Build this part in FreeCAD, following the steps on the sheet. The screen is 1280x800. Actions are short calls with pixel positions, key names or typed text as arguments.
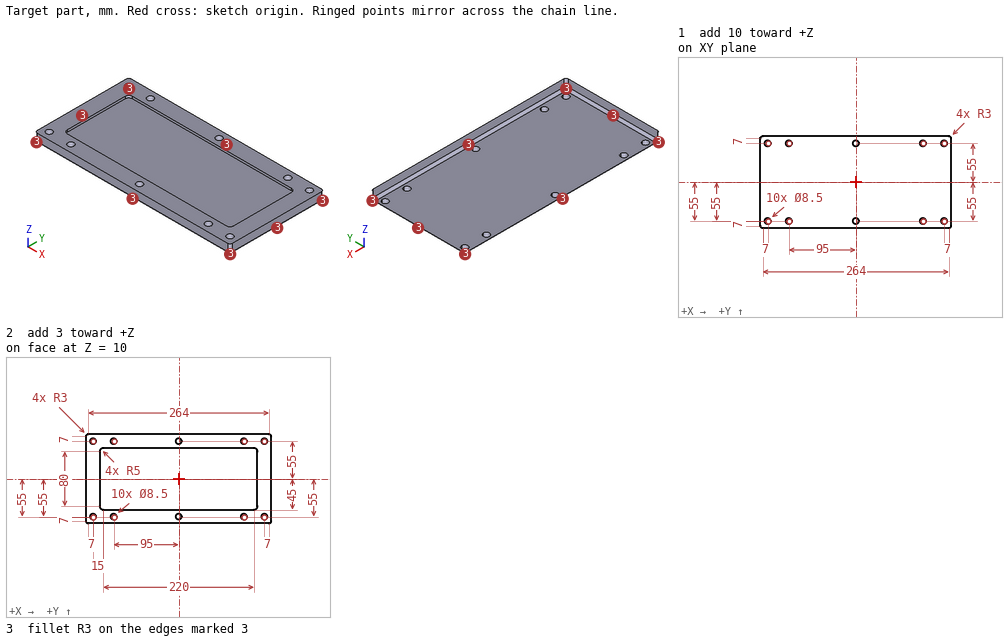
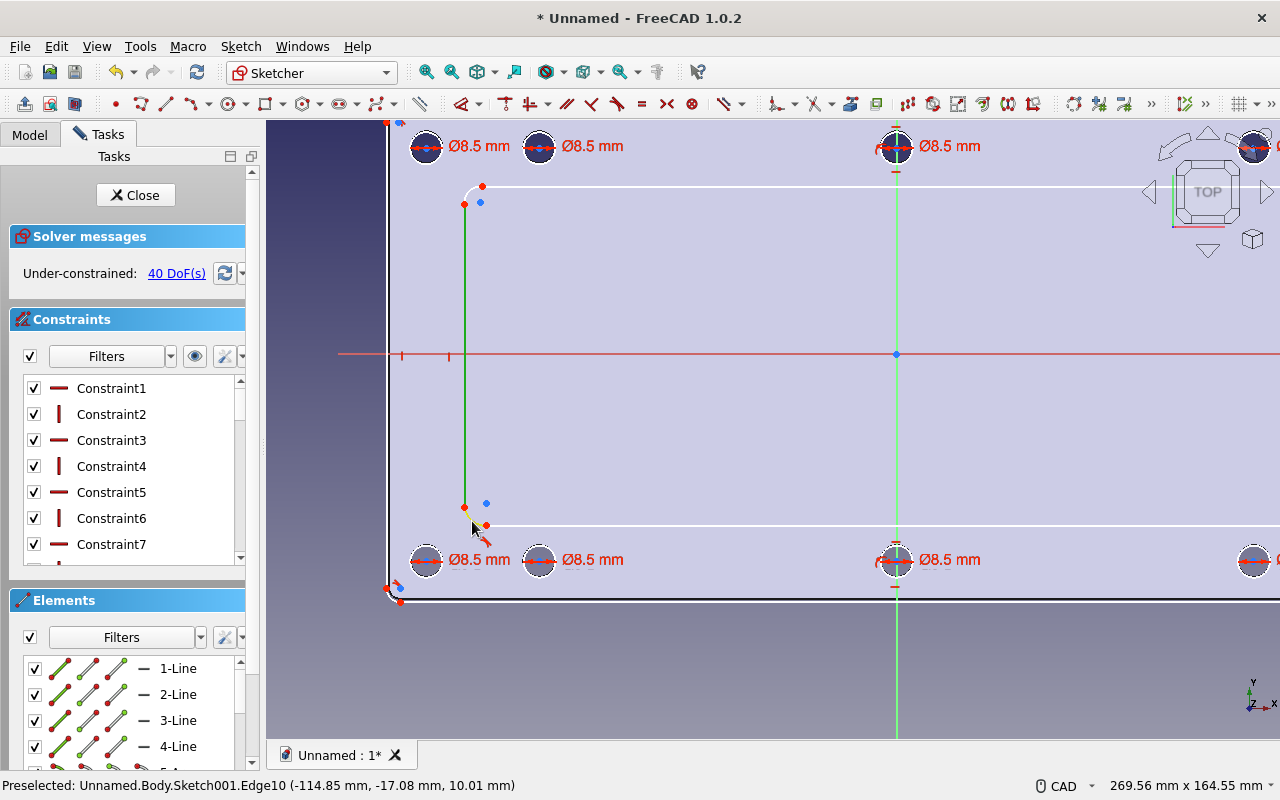
click(472, 521)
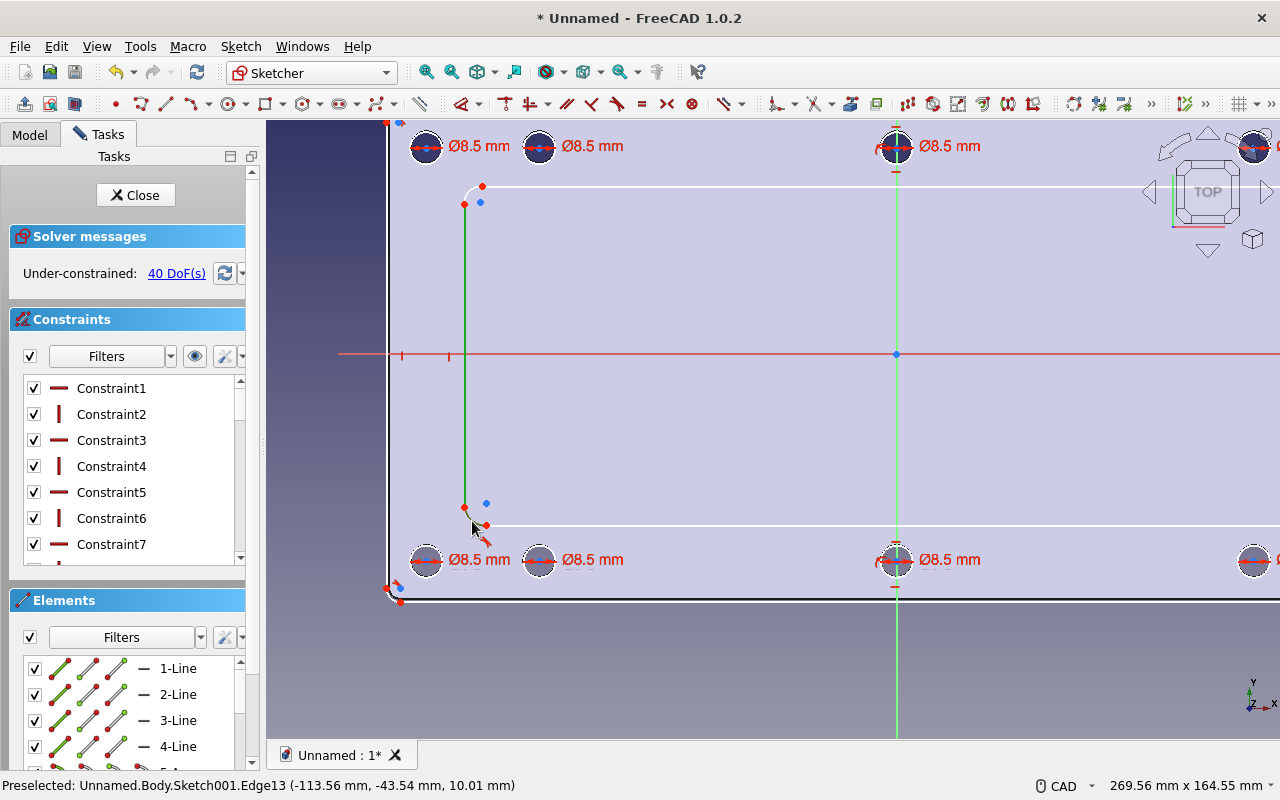
click(617, 104)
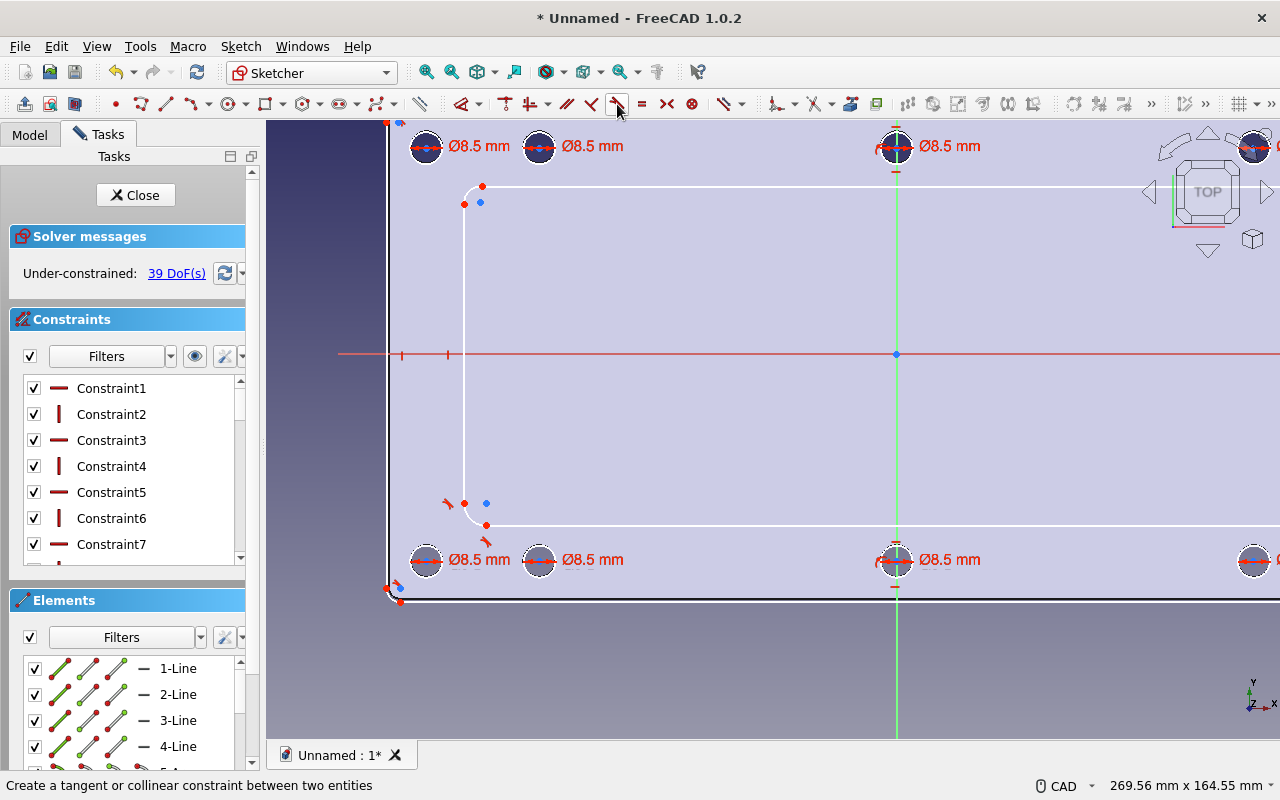
click(464, 414)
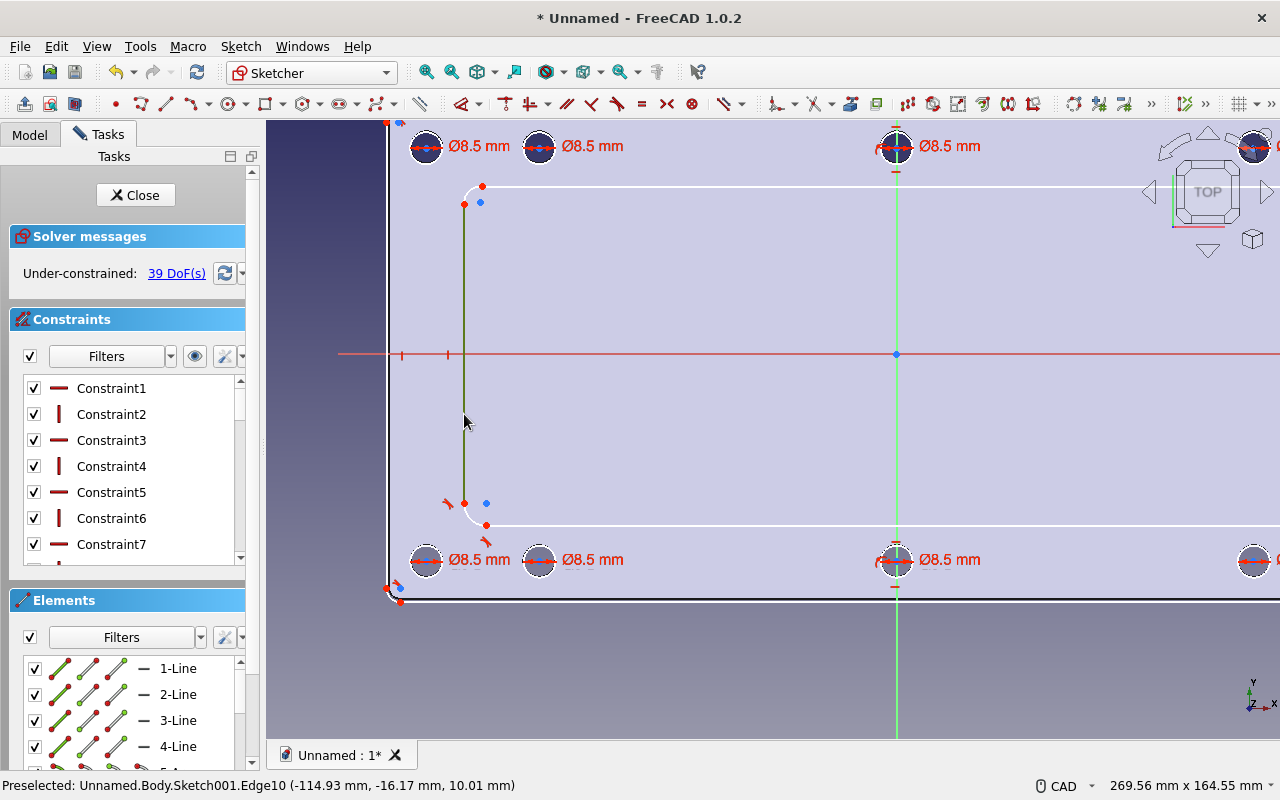
click(469, 191)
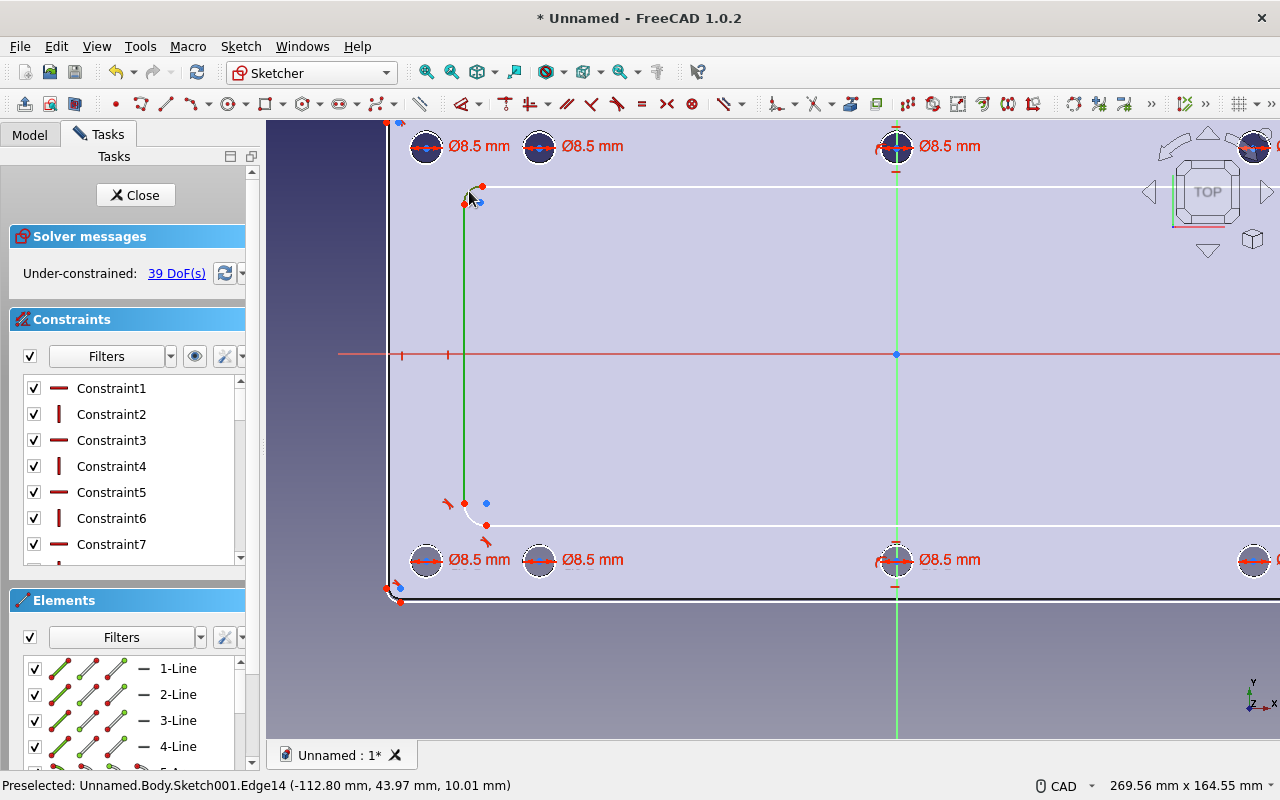
click(617, 104)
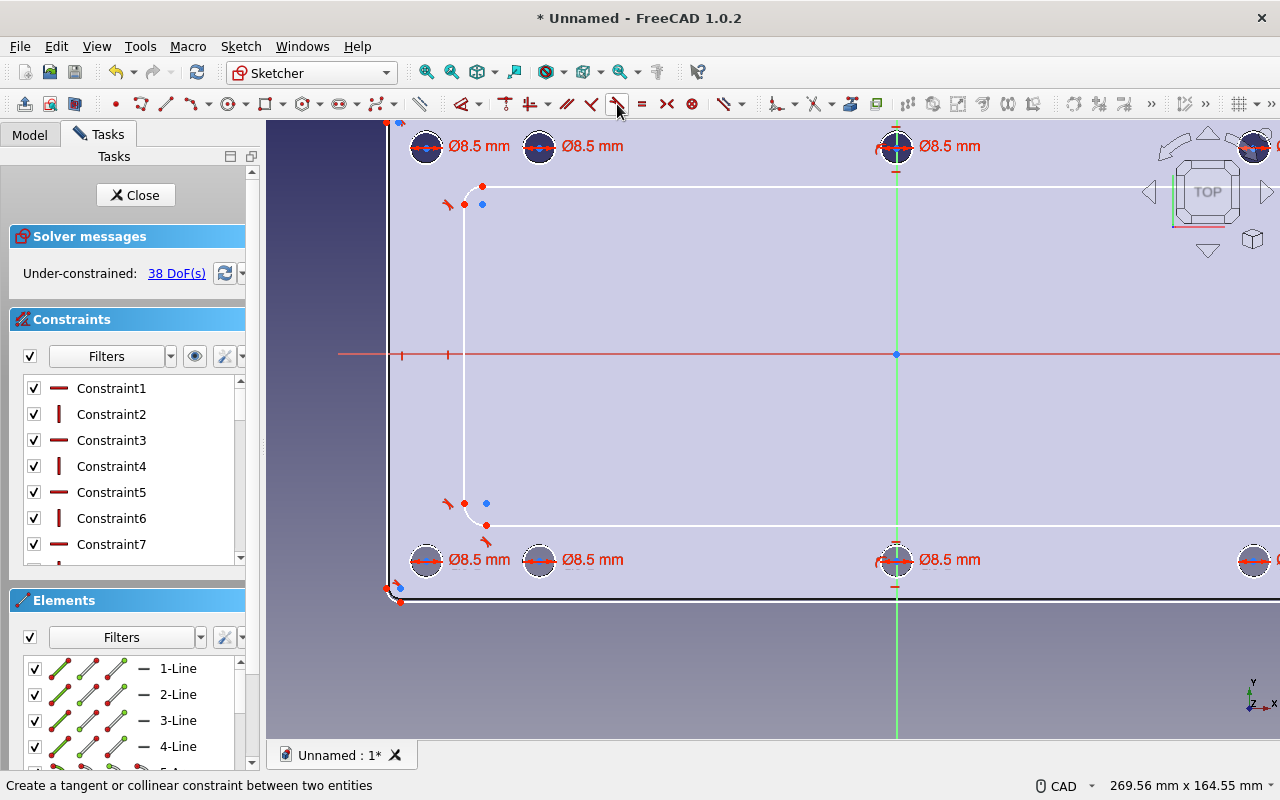
click(731, 187)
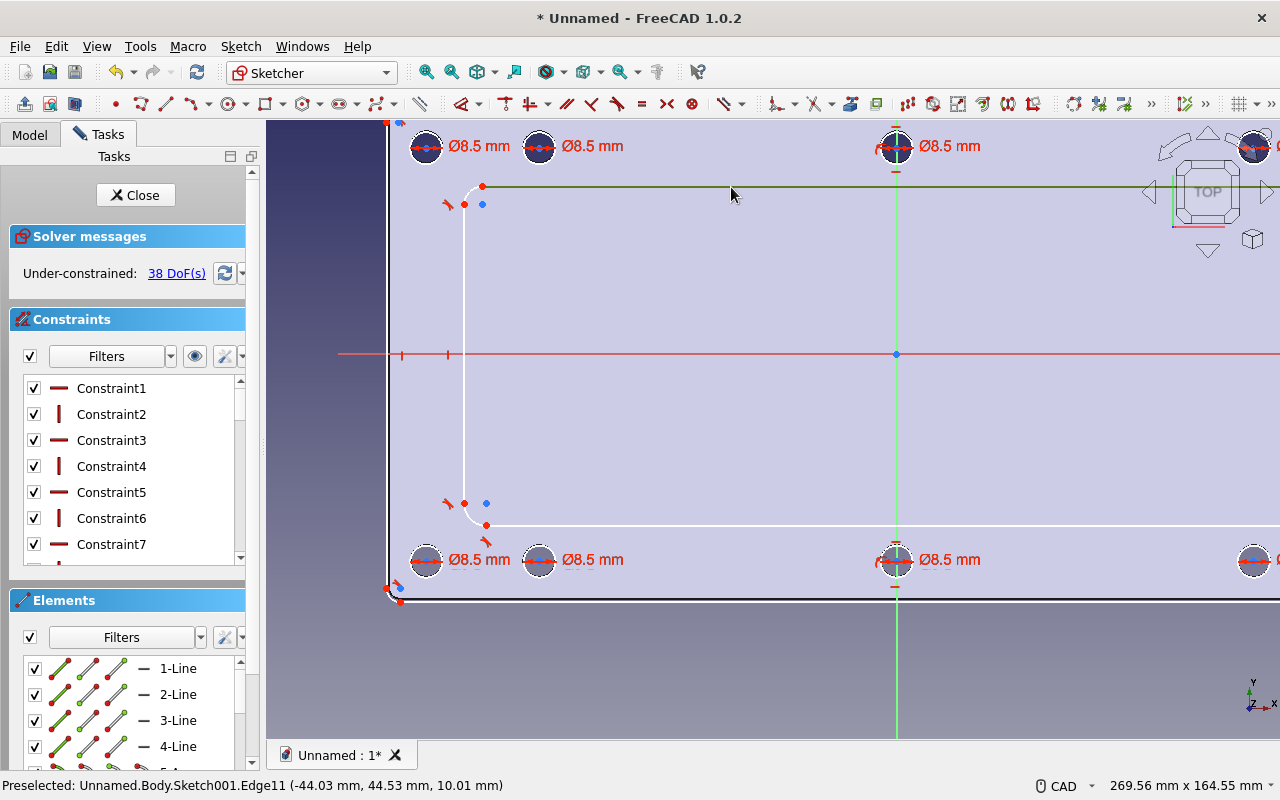
click(470, 192)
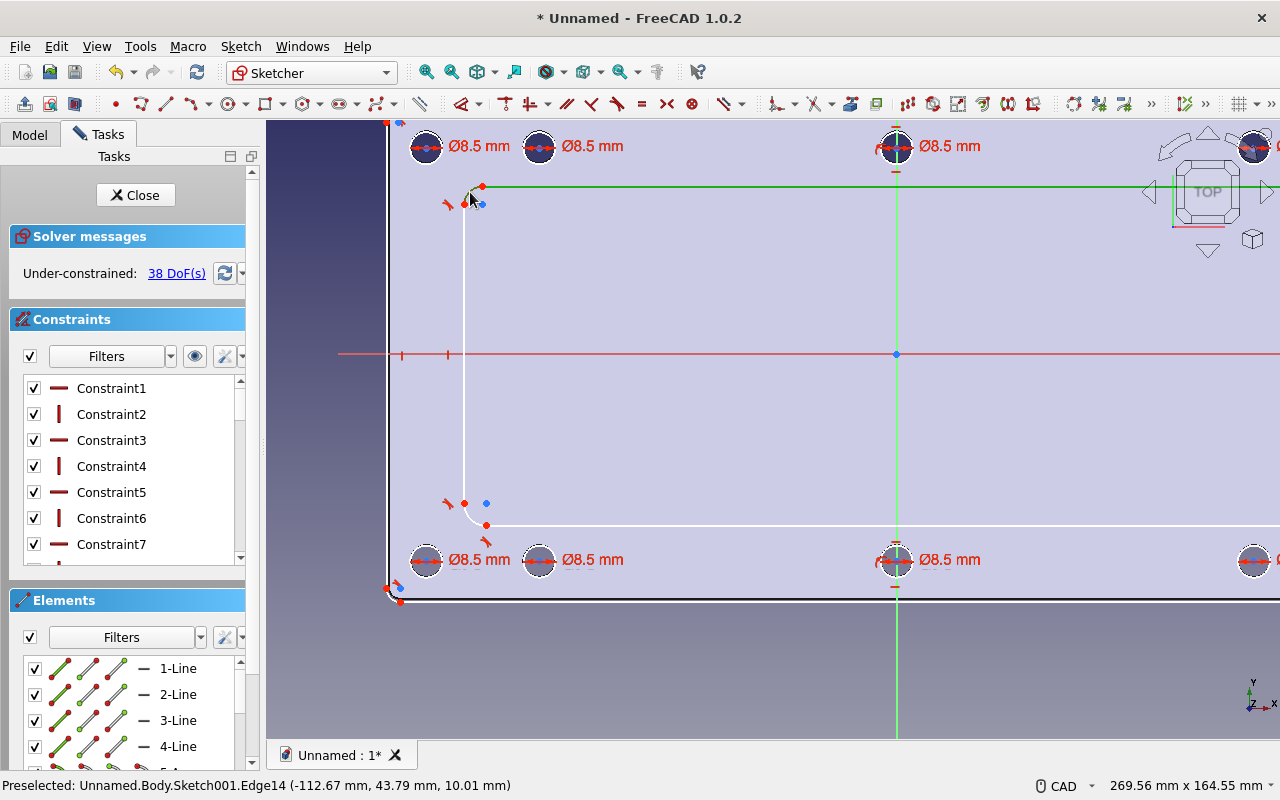
click(617, 104)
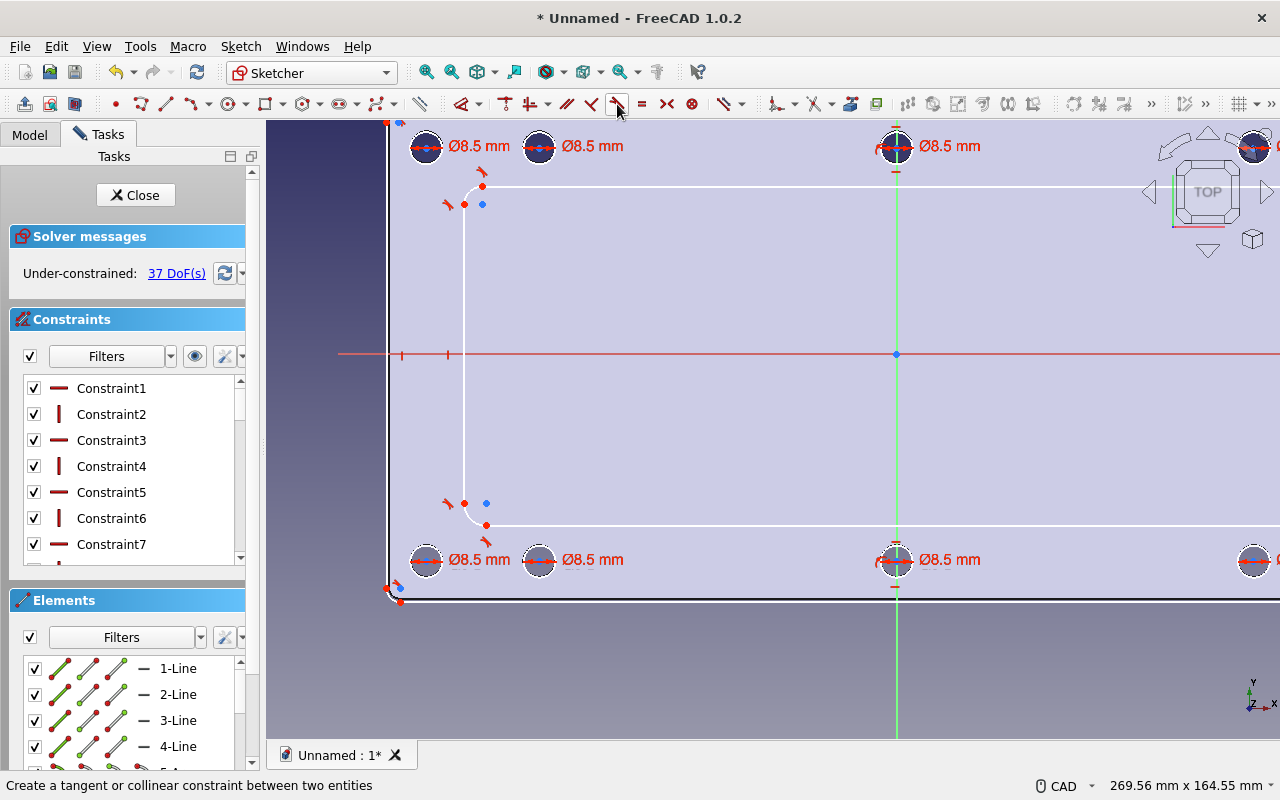
click(731, 187)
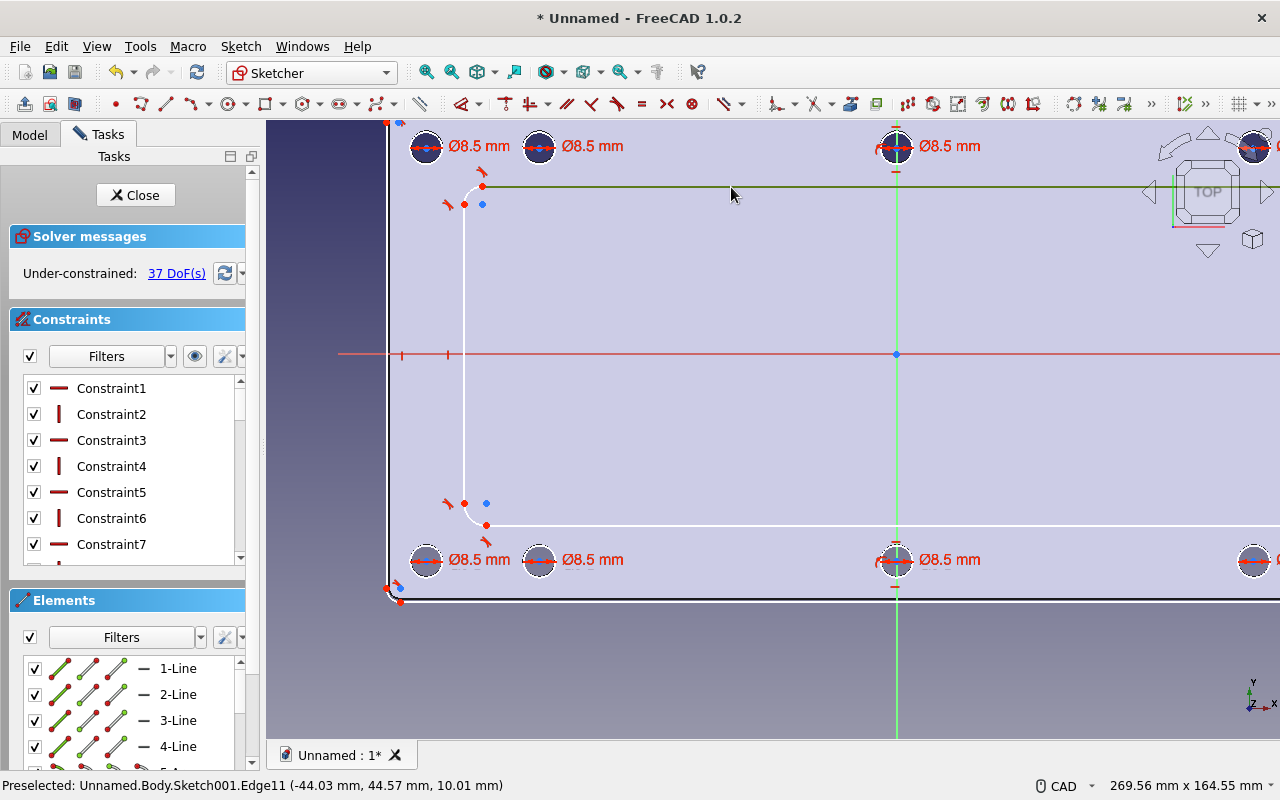
scroll(471, 521, down, 3)